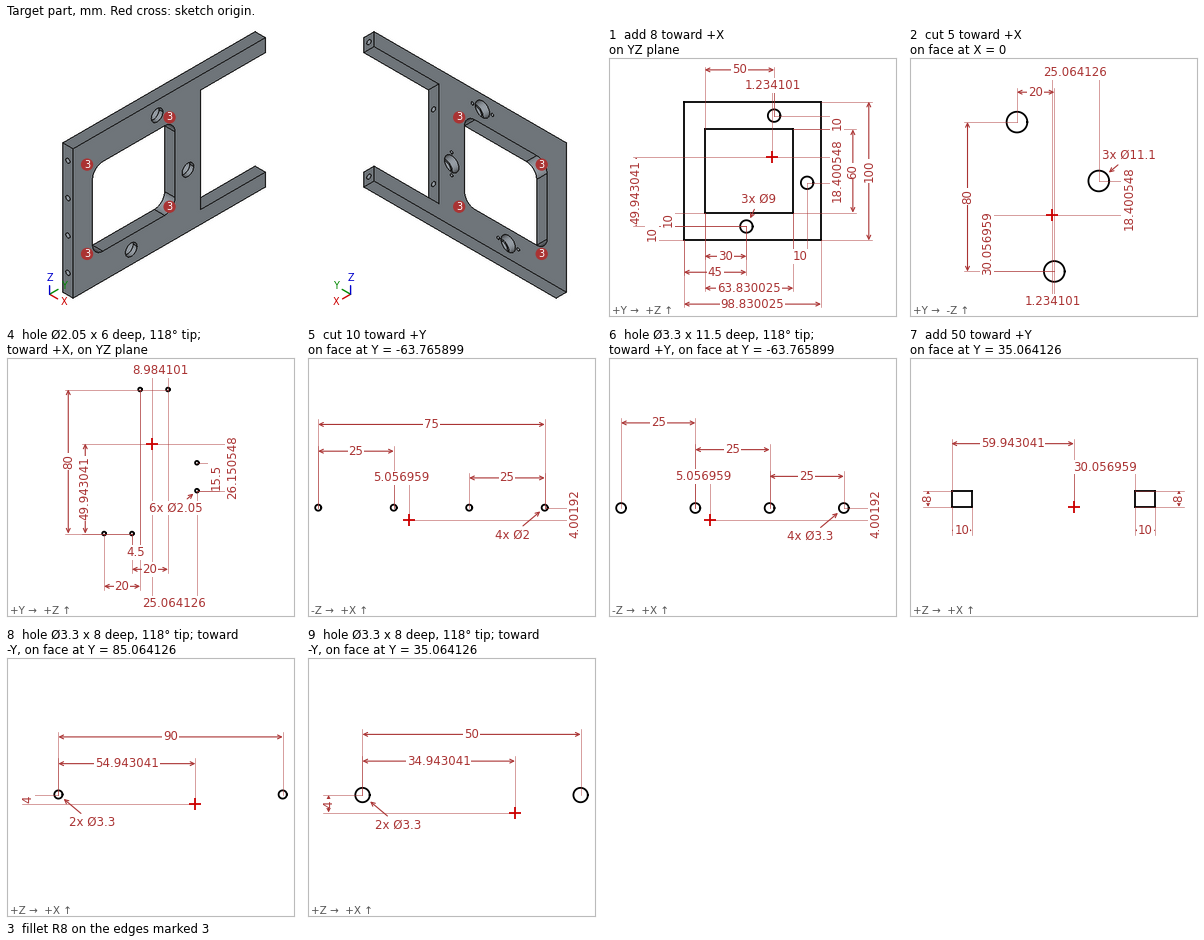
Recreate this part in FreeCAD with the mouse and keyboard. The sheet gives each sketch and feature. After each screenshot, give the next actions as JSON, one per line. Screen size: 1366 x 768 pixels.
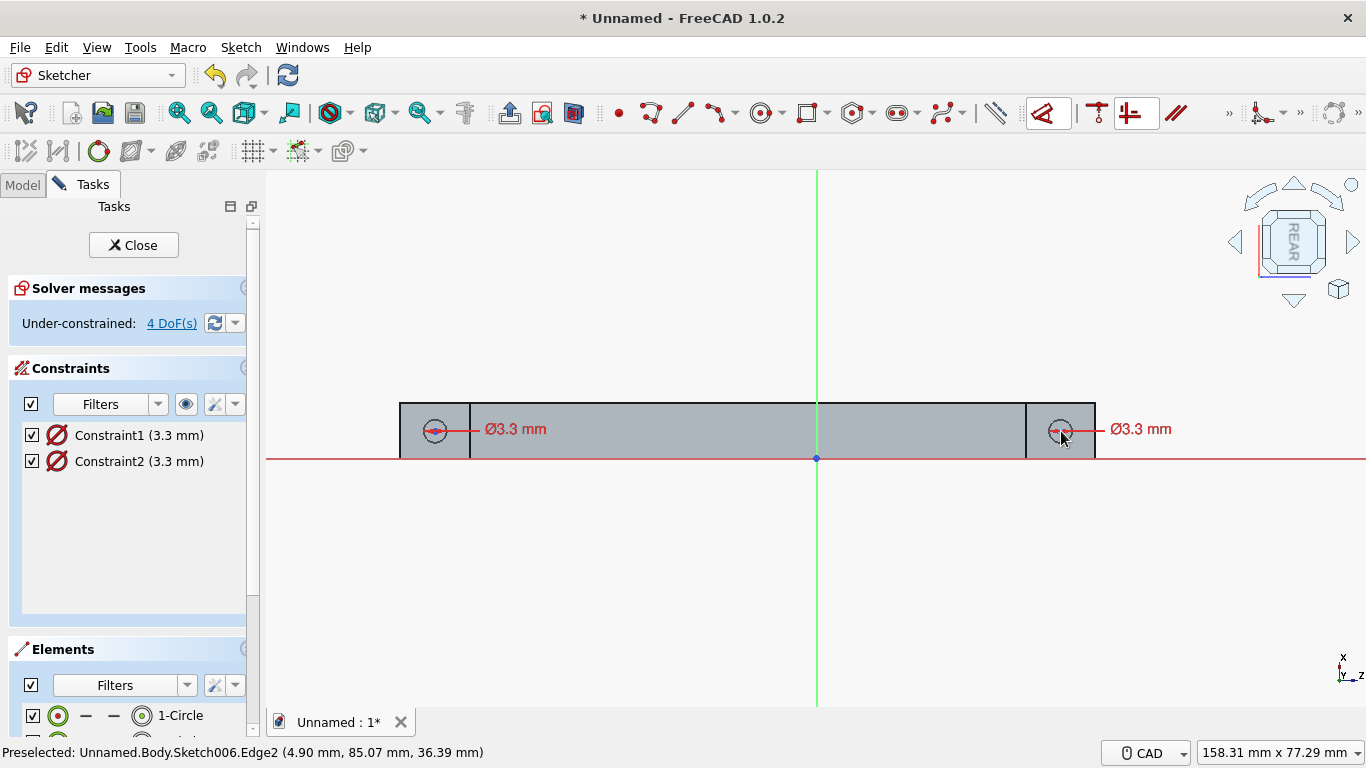
{"action": "left_click", "coordinate": [435, 431]}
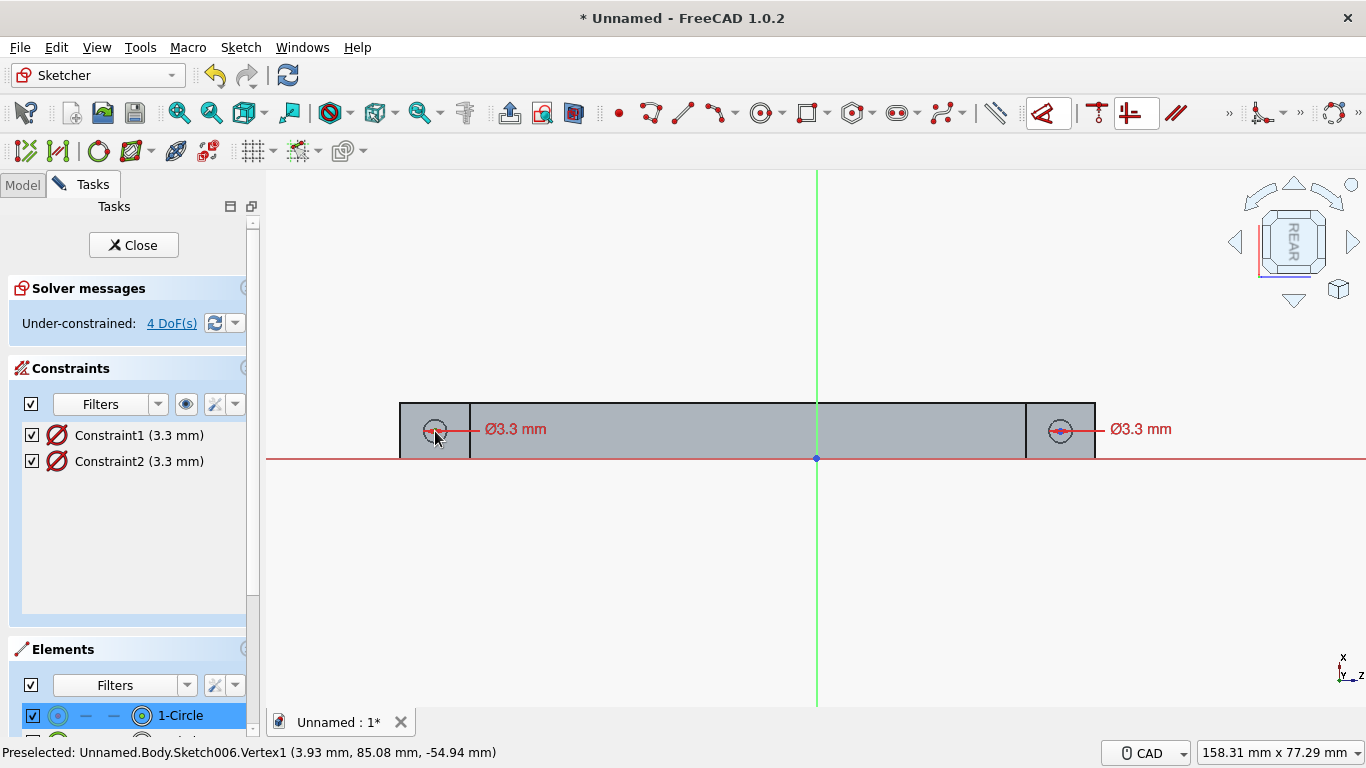
{"action": "left_click", "coordinate": [1060, 431]}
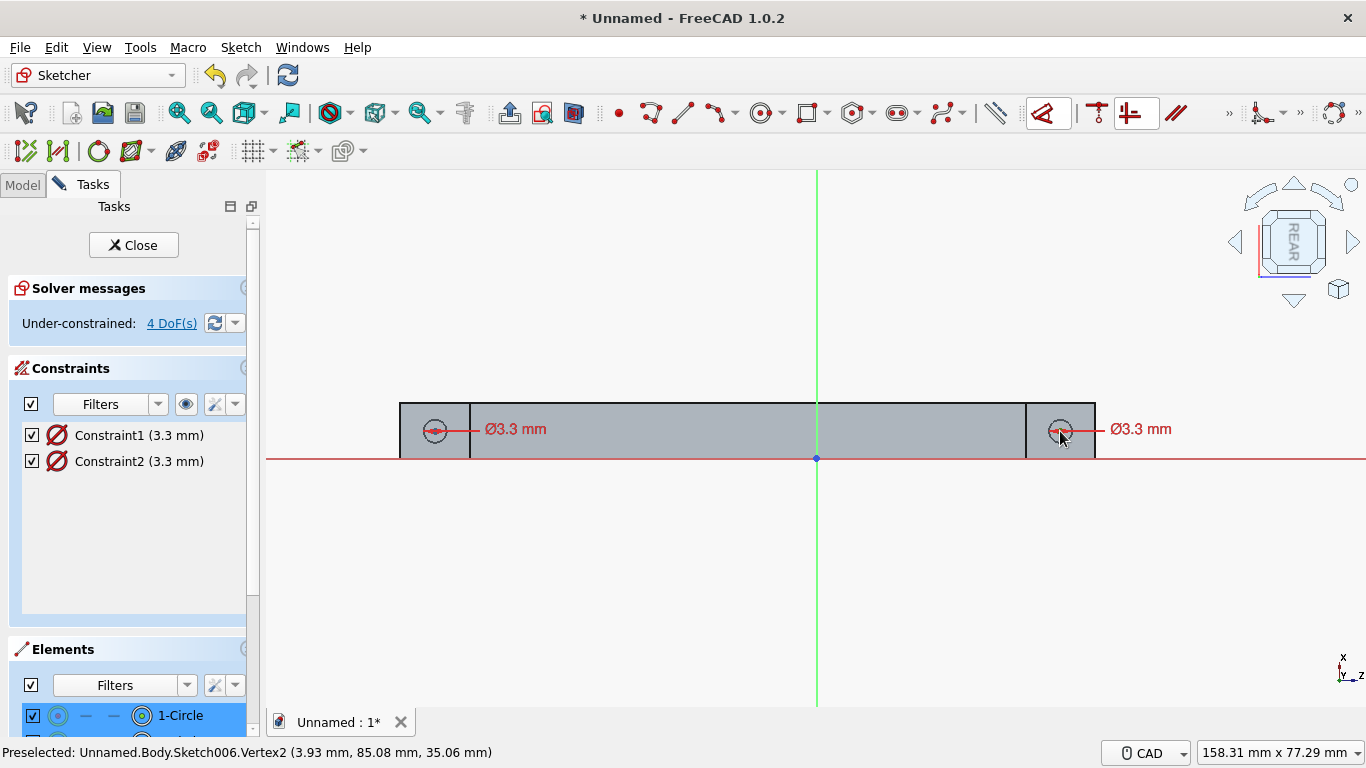
{"action": "left_click", "coordinate": [1154, 114]}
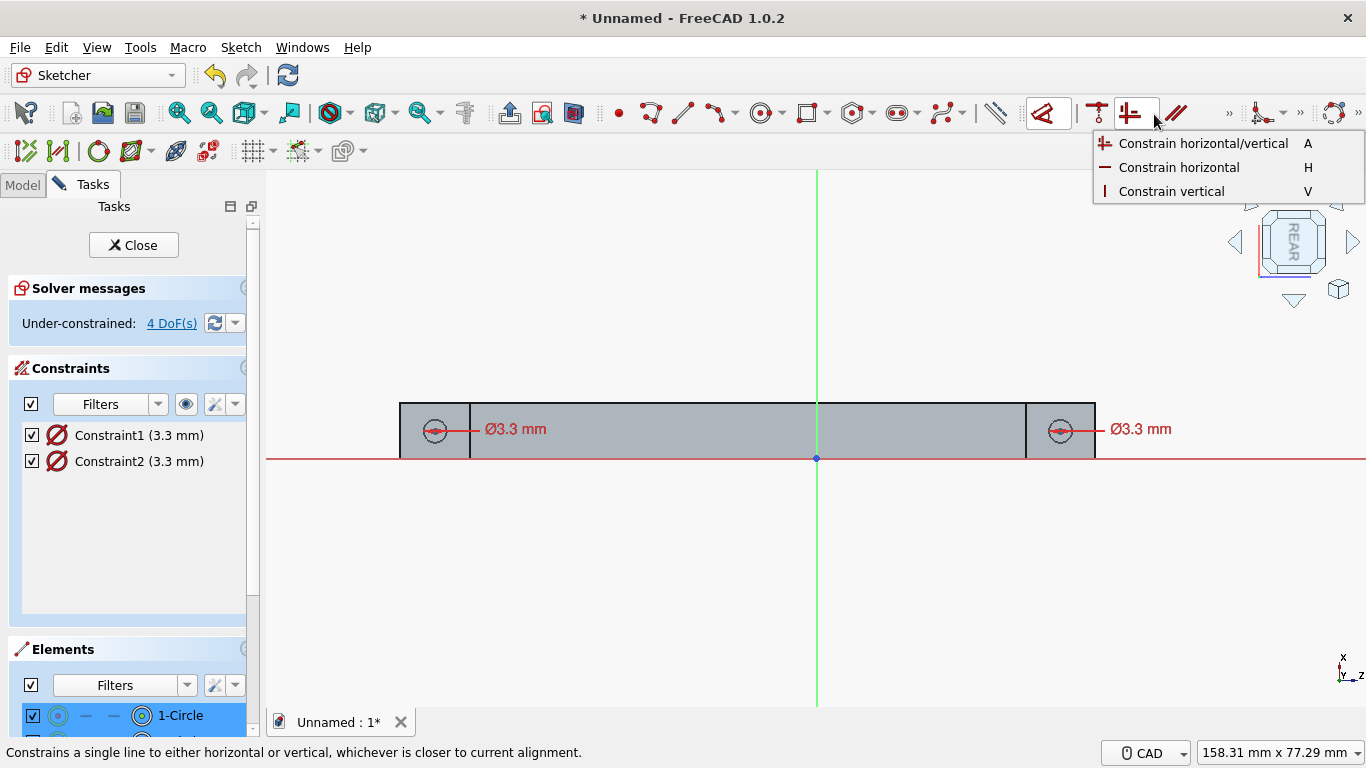
{"action": "left_click", "coordinate": [1229, 167]}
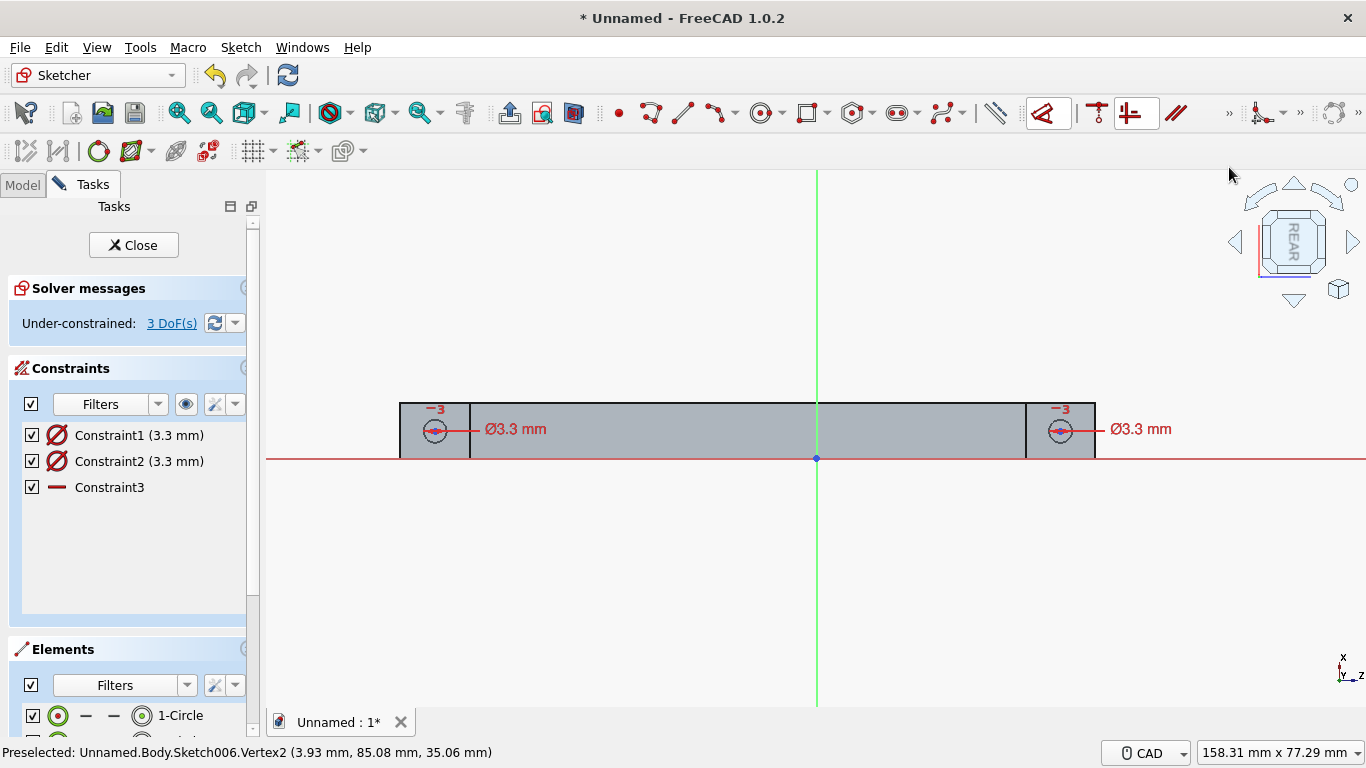
{"action": "scroll", "coordinate": [435, 431], "scroll_direction": "up", "scroll_amount": 2}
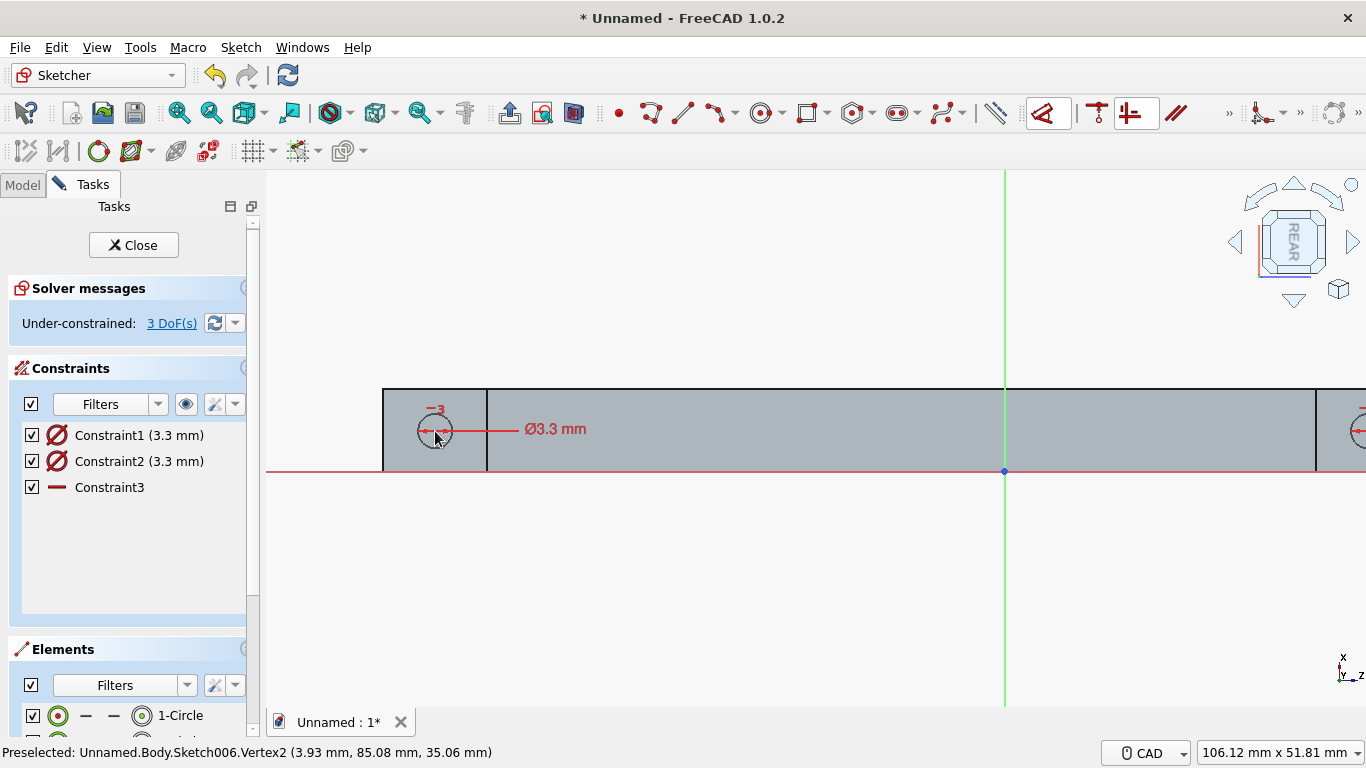
{"action": "left_click", "coordinate": [435, 431]}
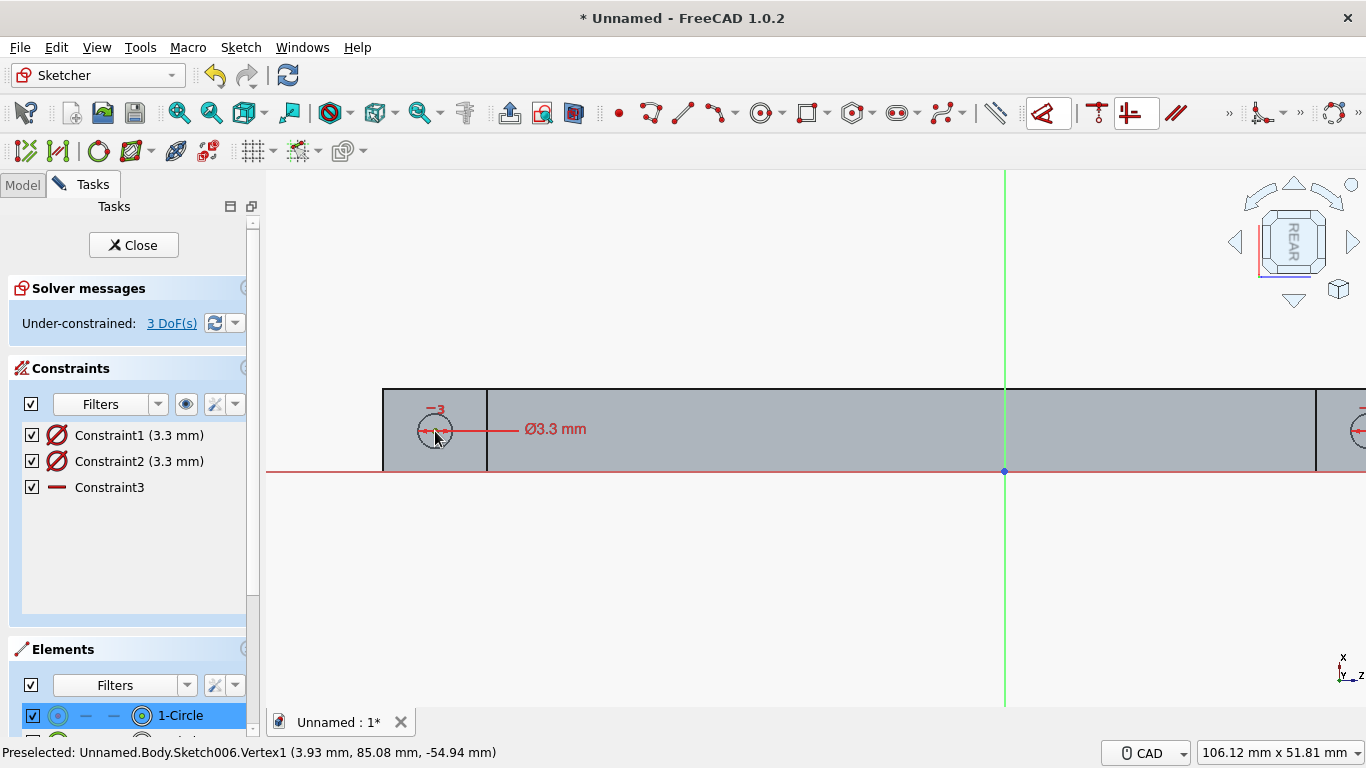
{"action": "left_click", "coordinate": [1066, 114]}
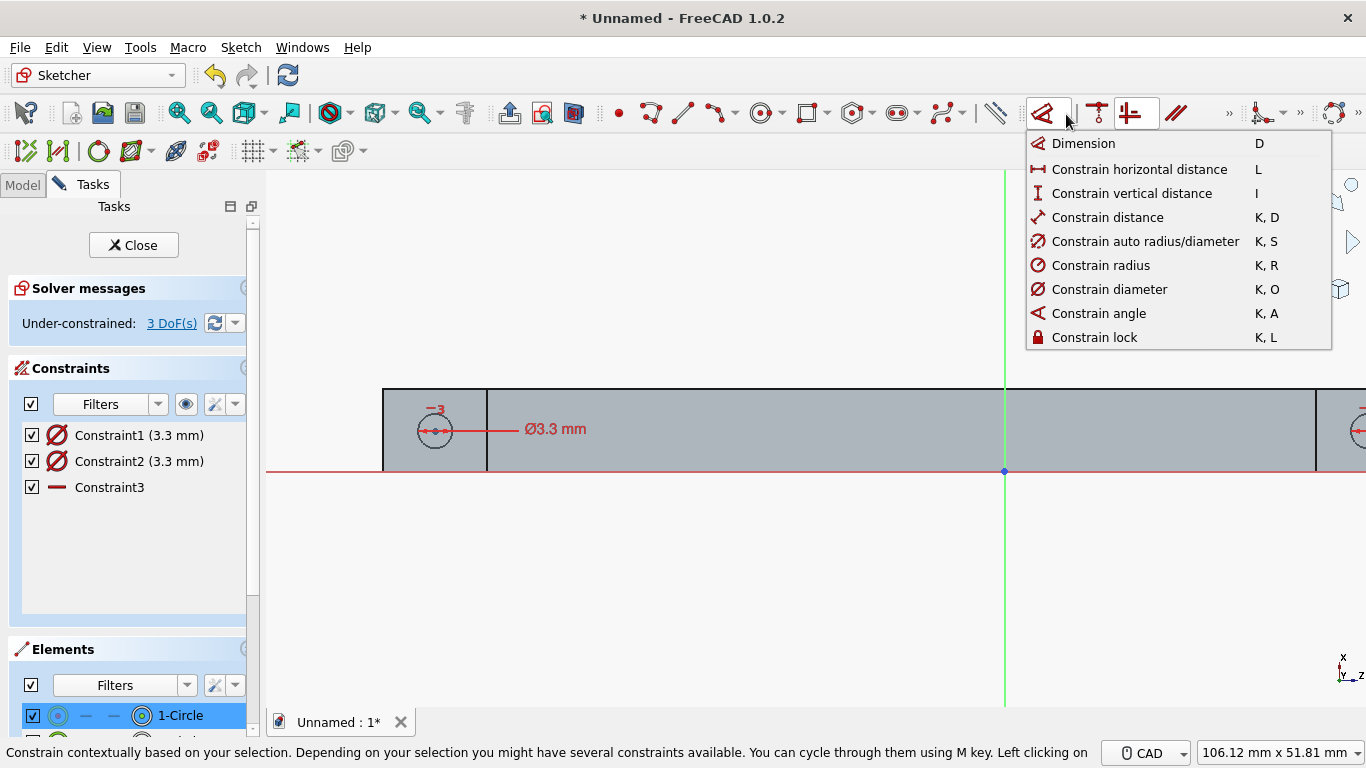
{"action": "left_click", "coordinate": [1179, 193]}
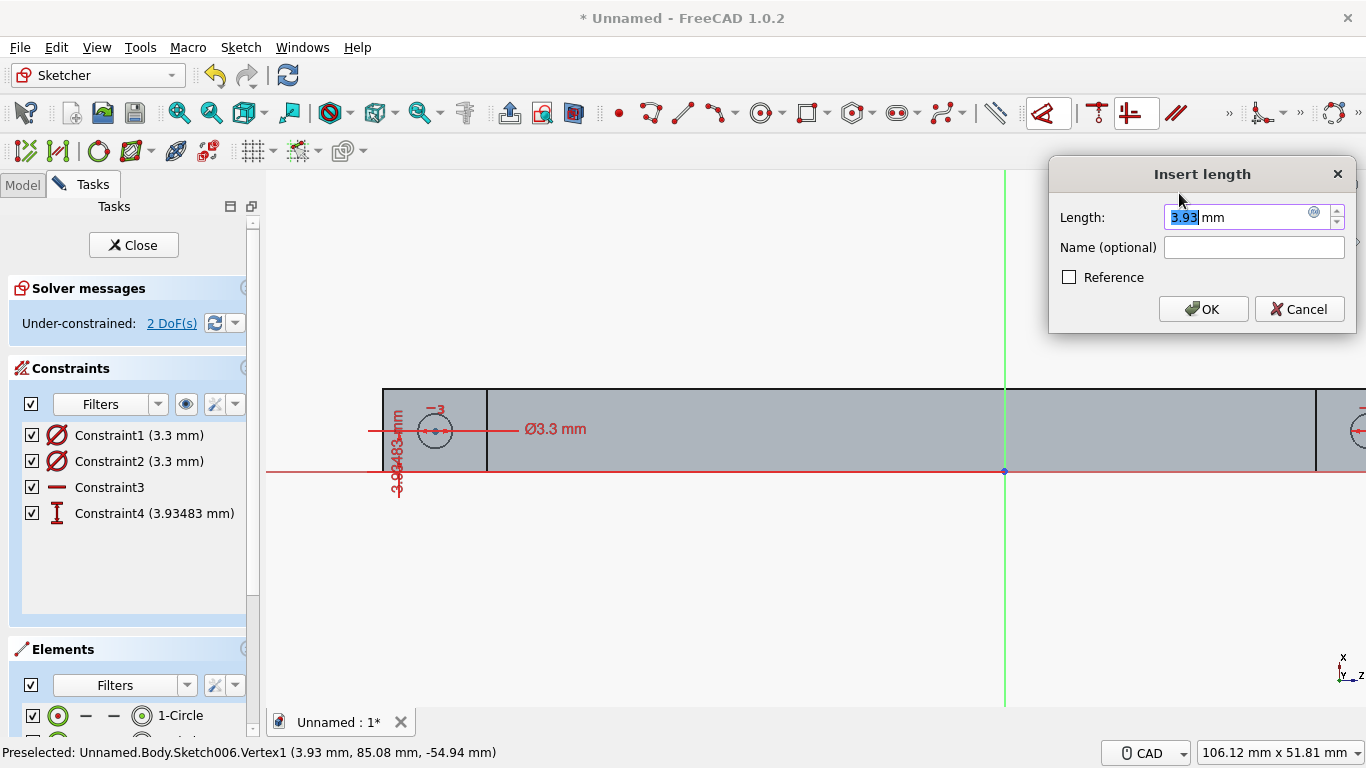
{"action": "type", "text": "4"}
{"action": "key", "text": "Return"}